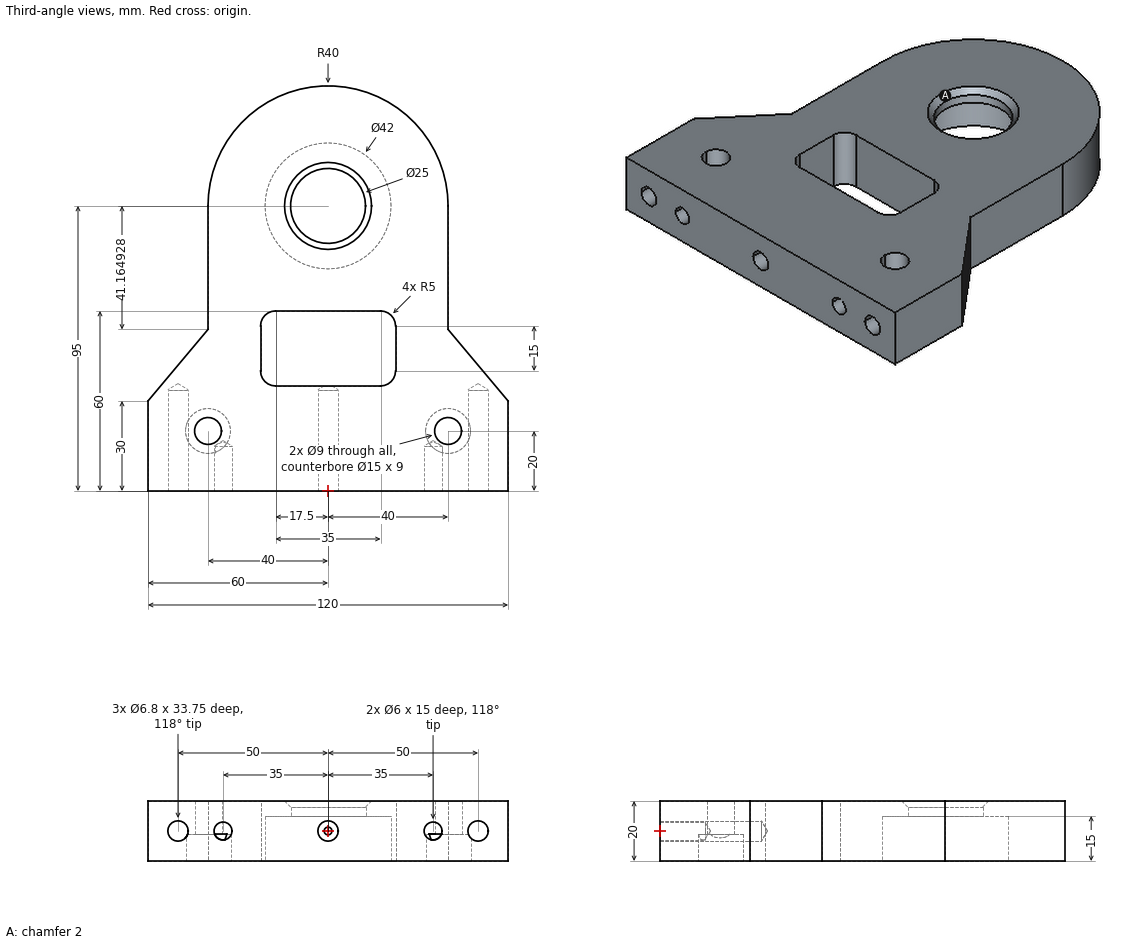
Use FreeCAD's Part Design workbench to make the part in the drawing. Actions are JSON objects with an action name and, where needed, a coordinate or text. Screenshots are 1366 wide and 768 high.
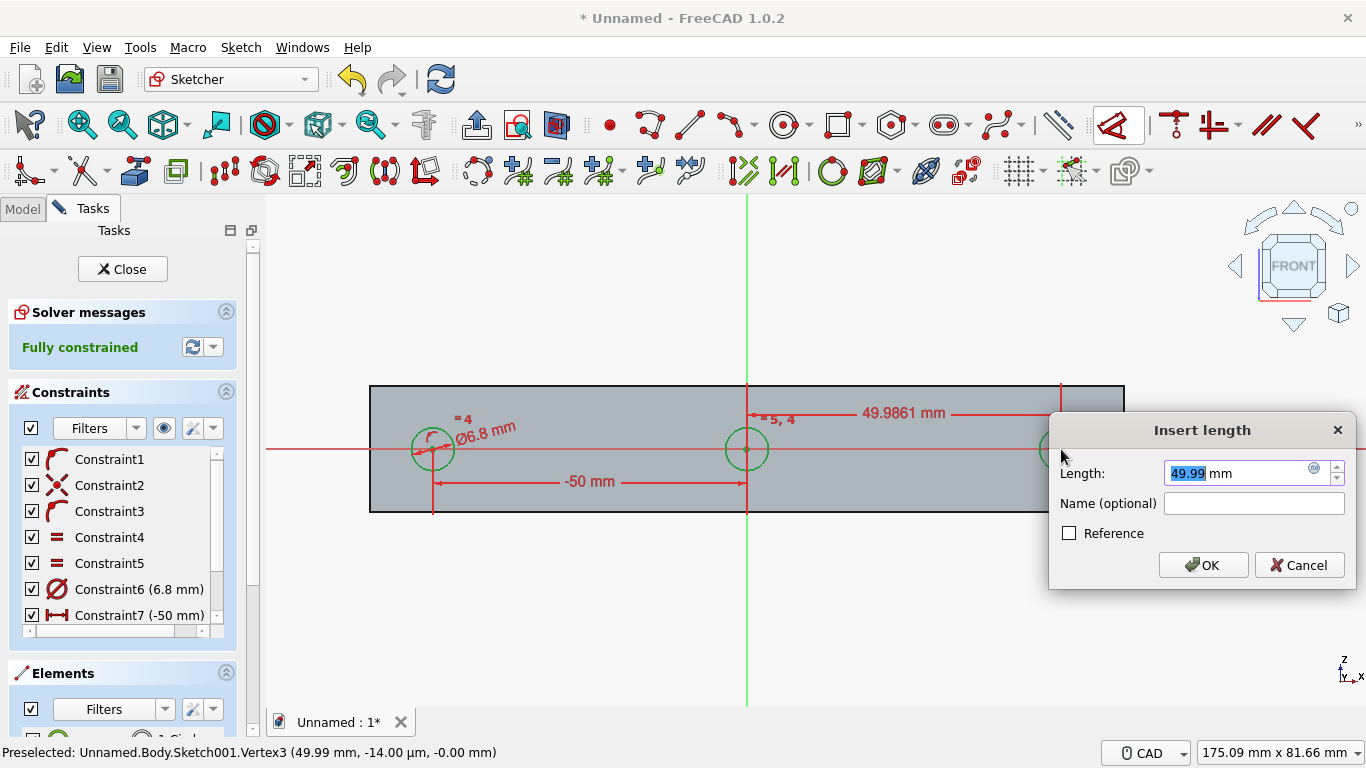
{"action": "type", "text": "50"}
{"action": "key", "text": "Return"}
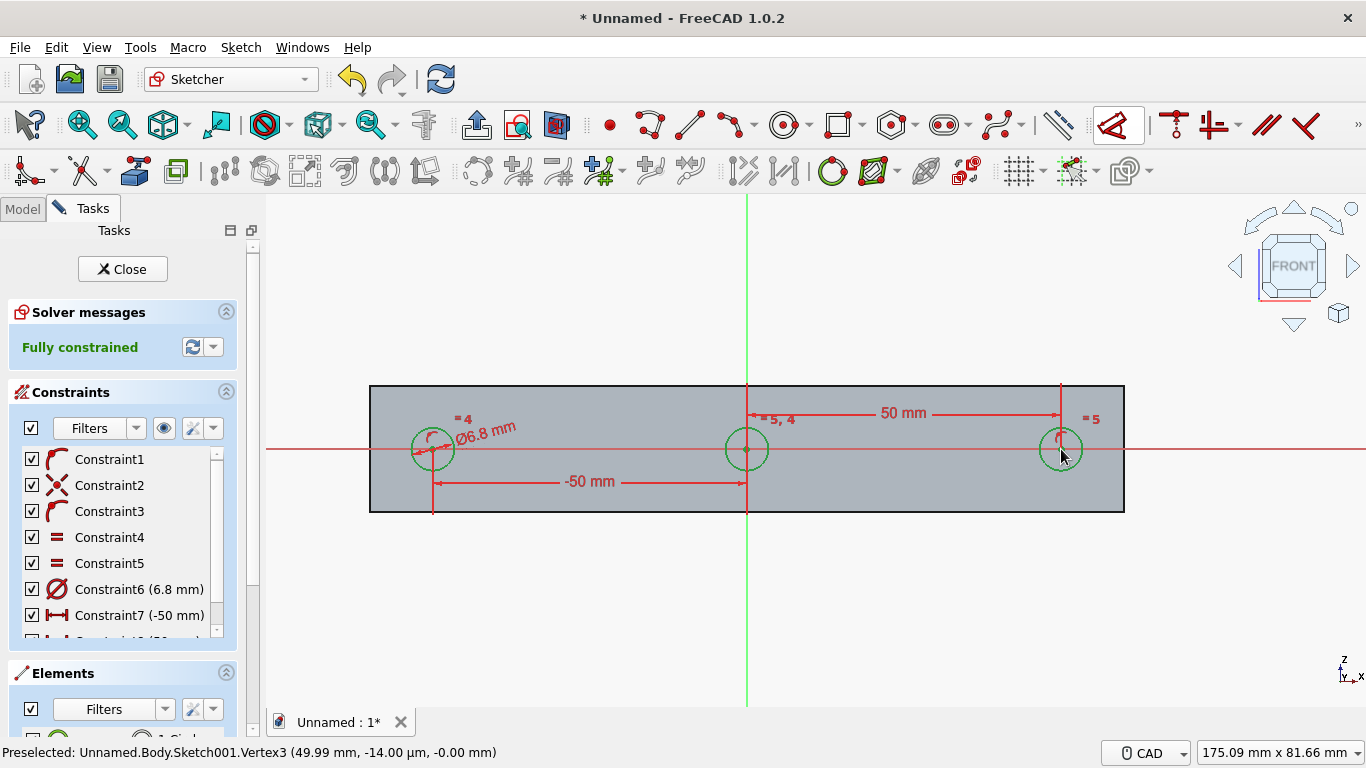
{"action": "left_click", "coordinate": [123, 269]}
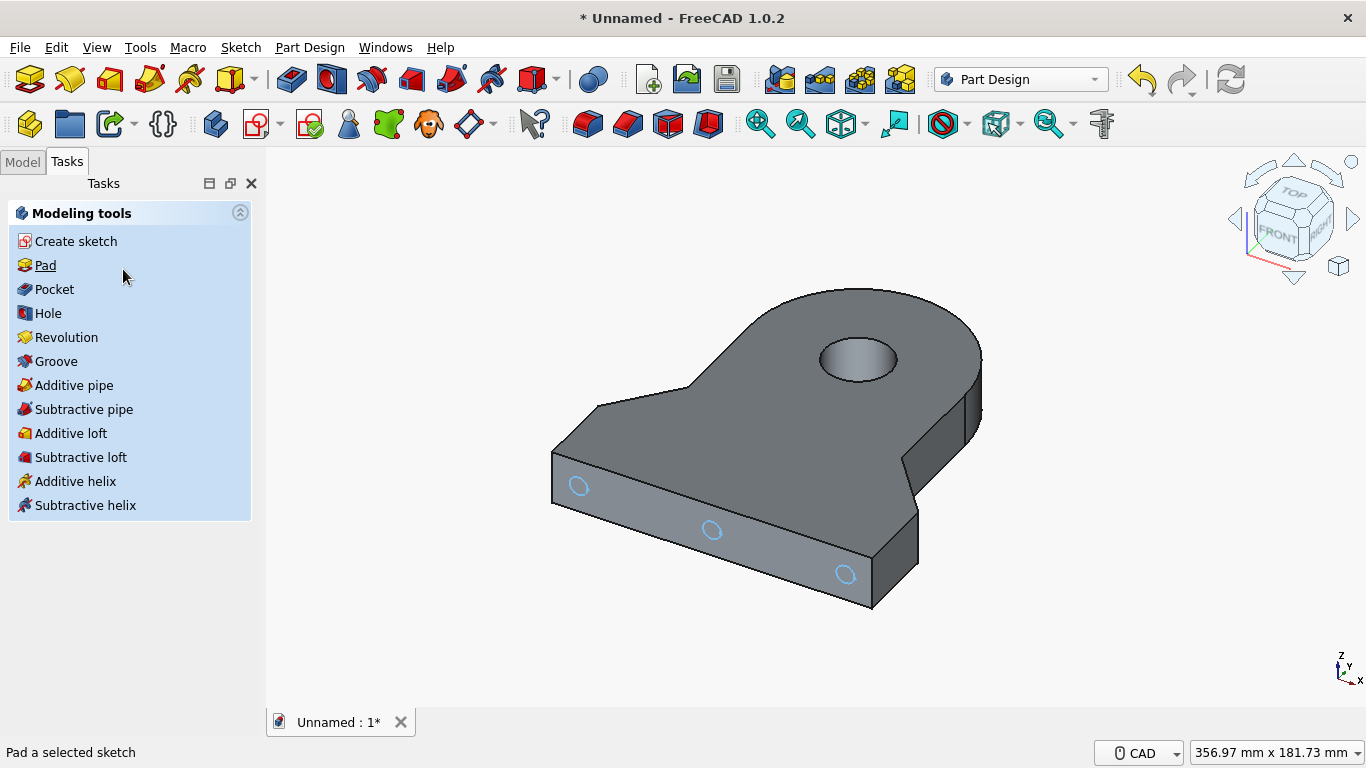
{"action": "left_click", "coordinate": [332, 80]}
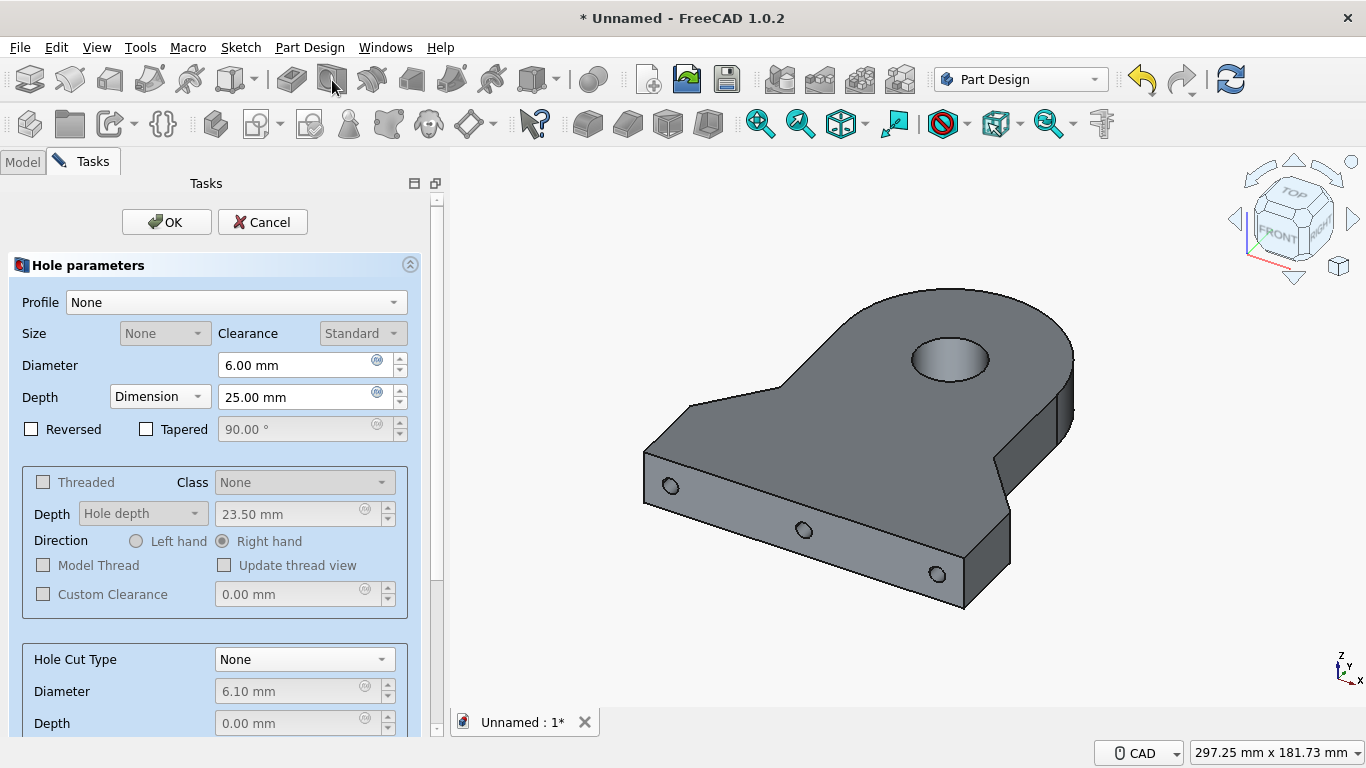
{"action": "triple_click", "coordinate": [305, 365]}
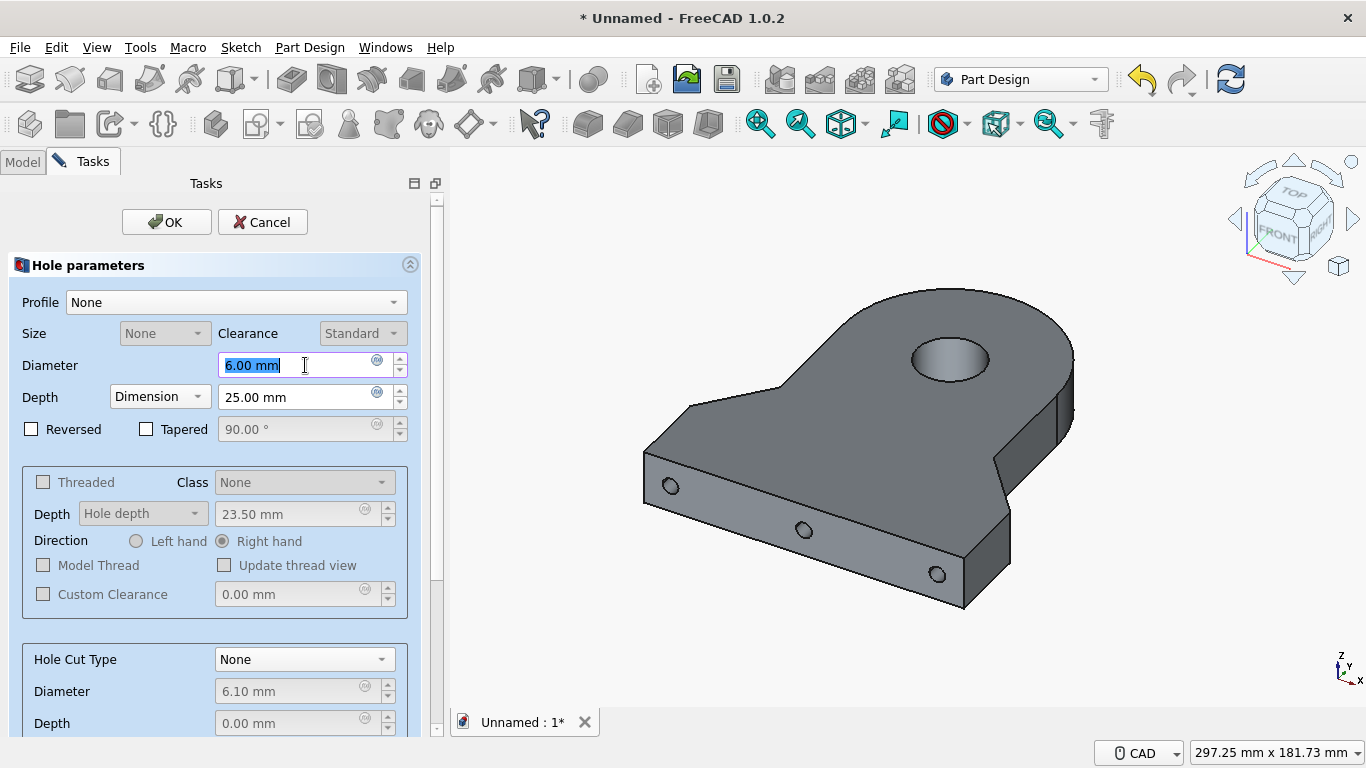
{"action": "type", "text": "6.8"}
{"action": "key", "text": "Tab"}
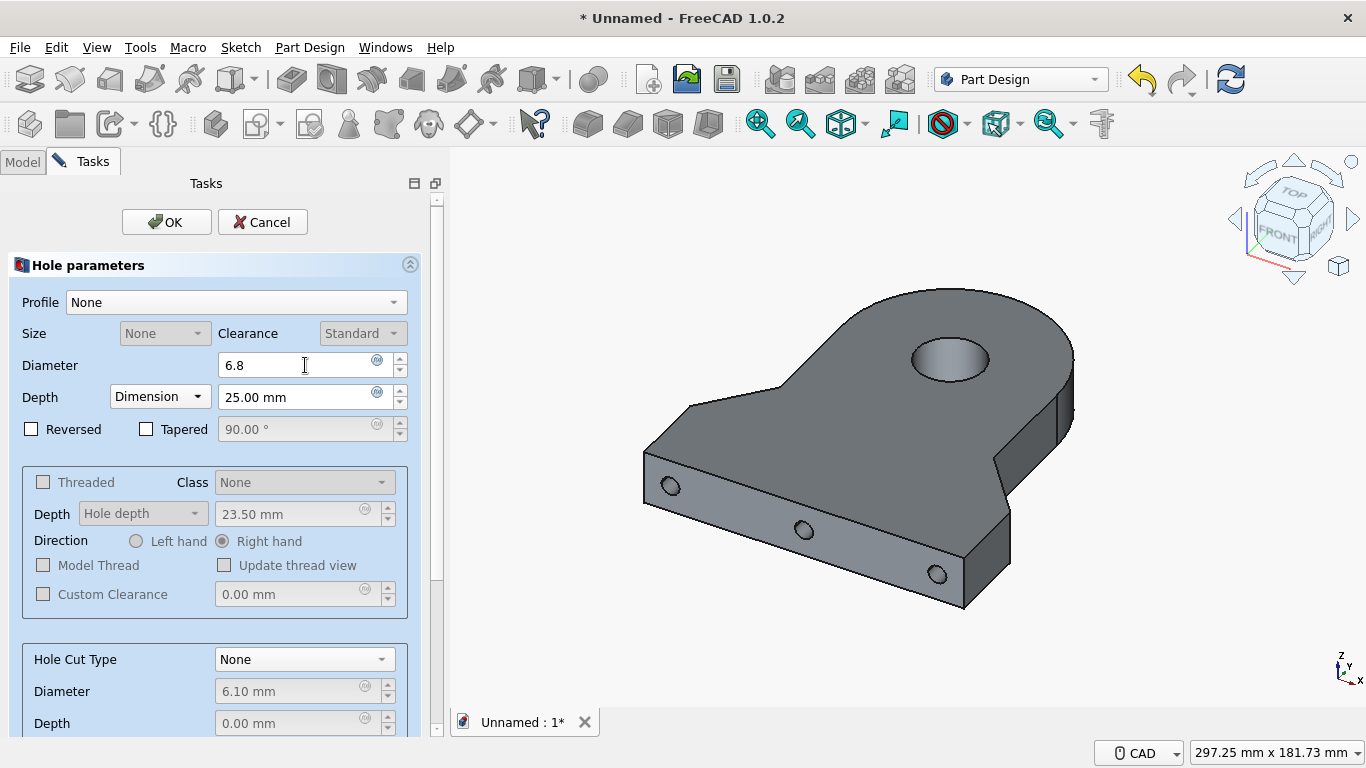
{"action": "triple_click", "coordinate": [305, 397]}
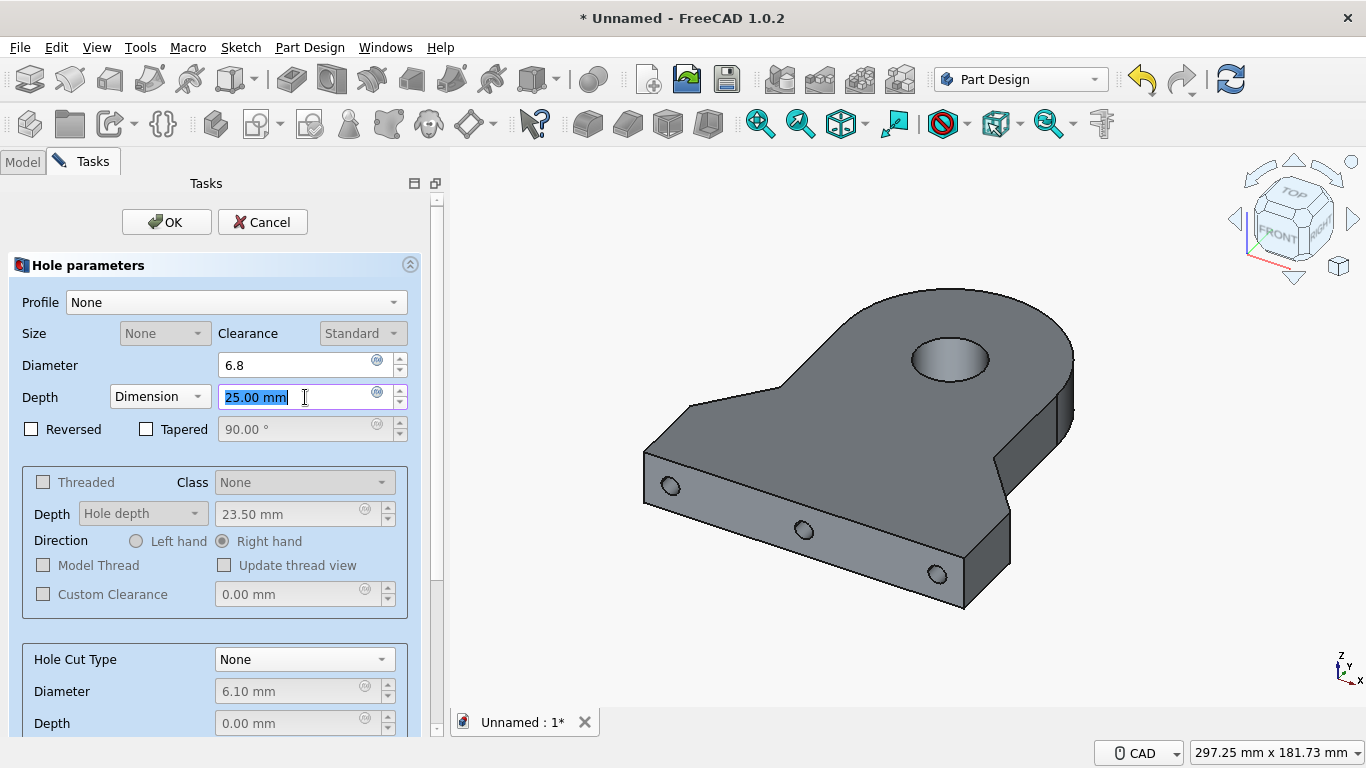
{"action": "type", "text": "33.75"}
{"action": "key", "text": "Tab"}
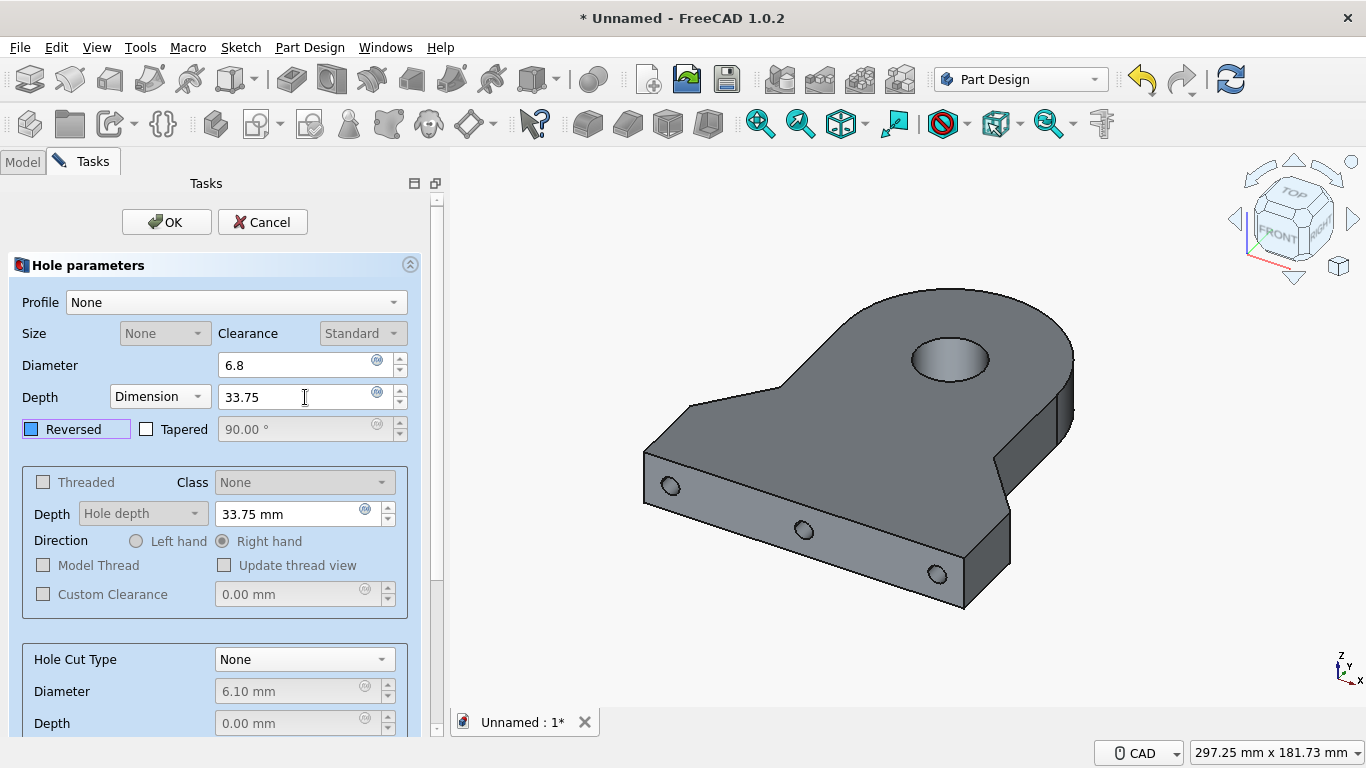
{"action": "left_click", "coordinate": [167, 222]}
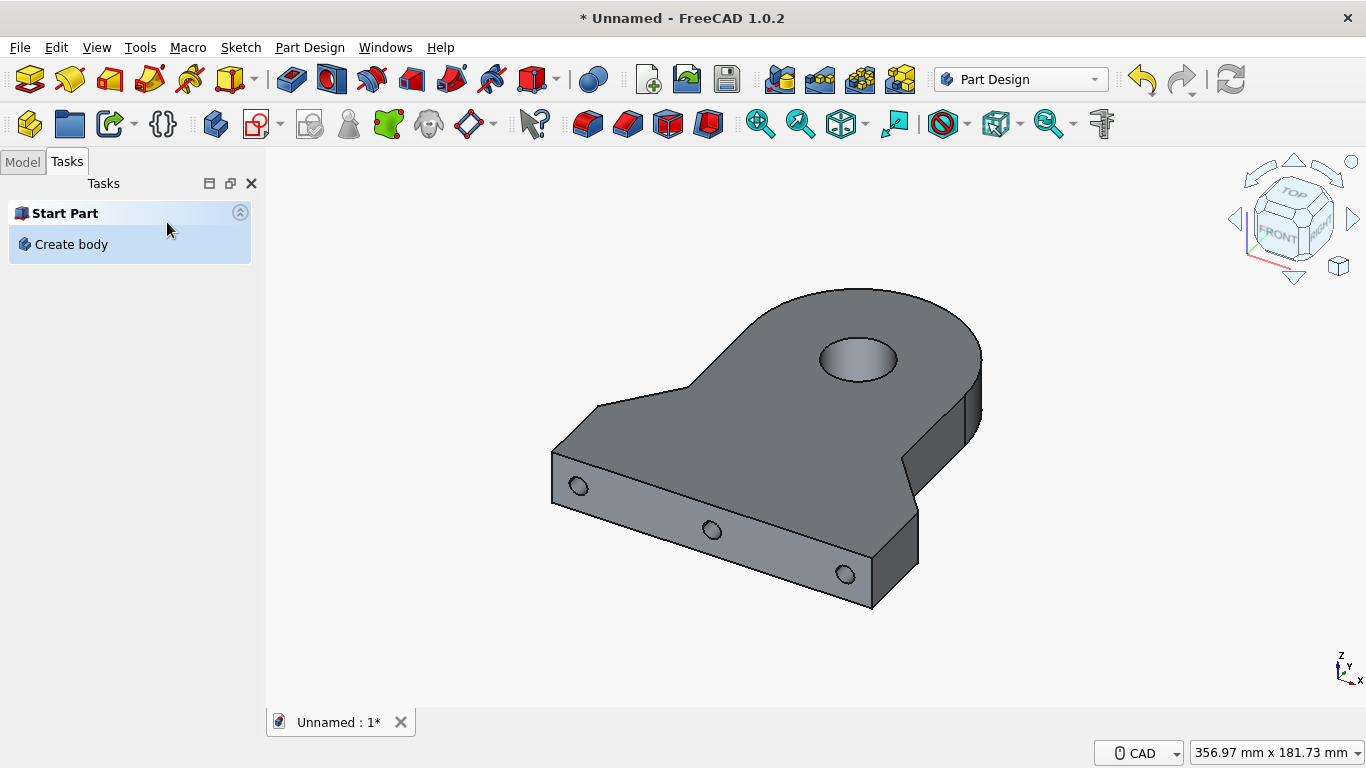
{"action": "left_click", "coordinate": [803, 560]}